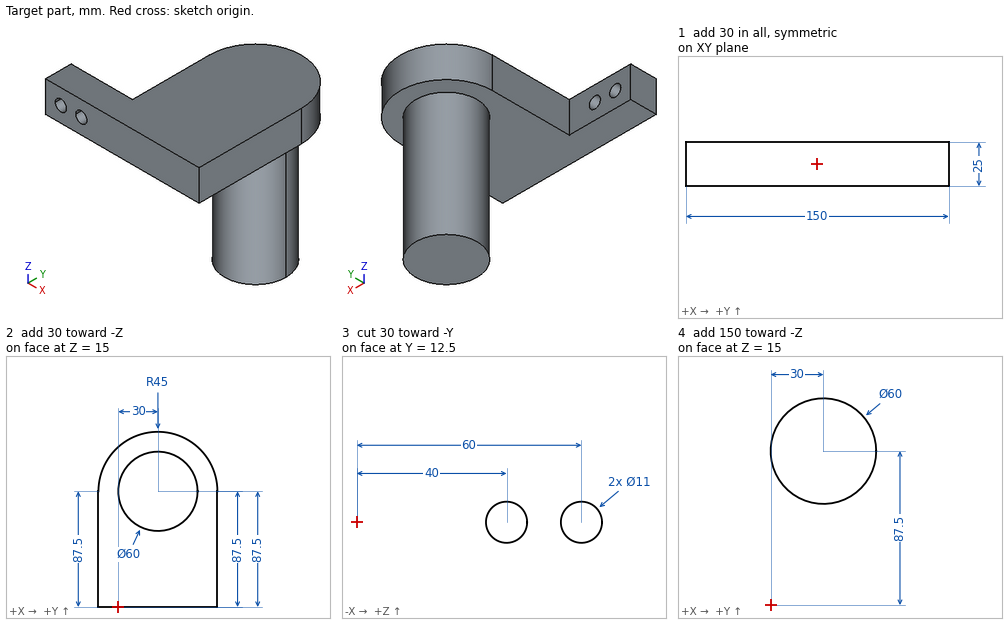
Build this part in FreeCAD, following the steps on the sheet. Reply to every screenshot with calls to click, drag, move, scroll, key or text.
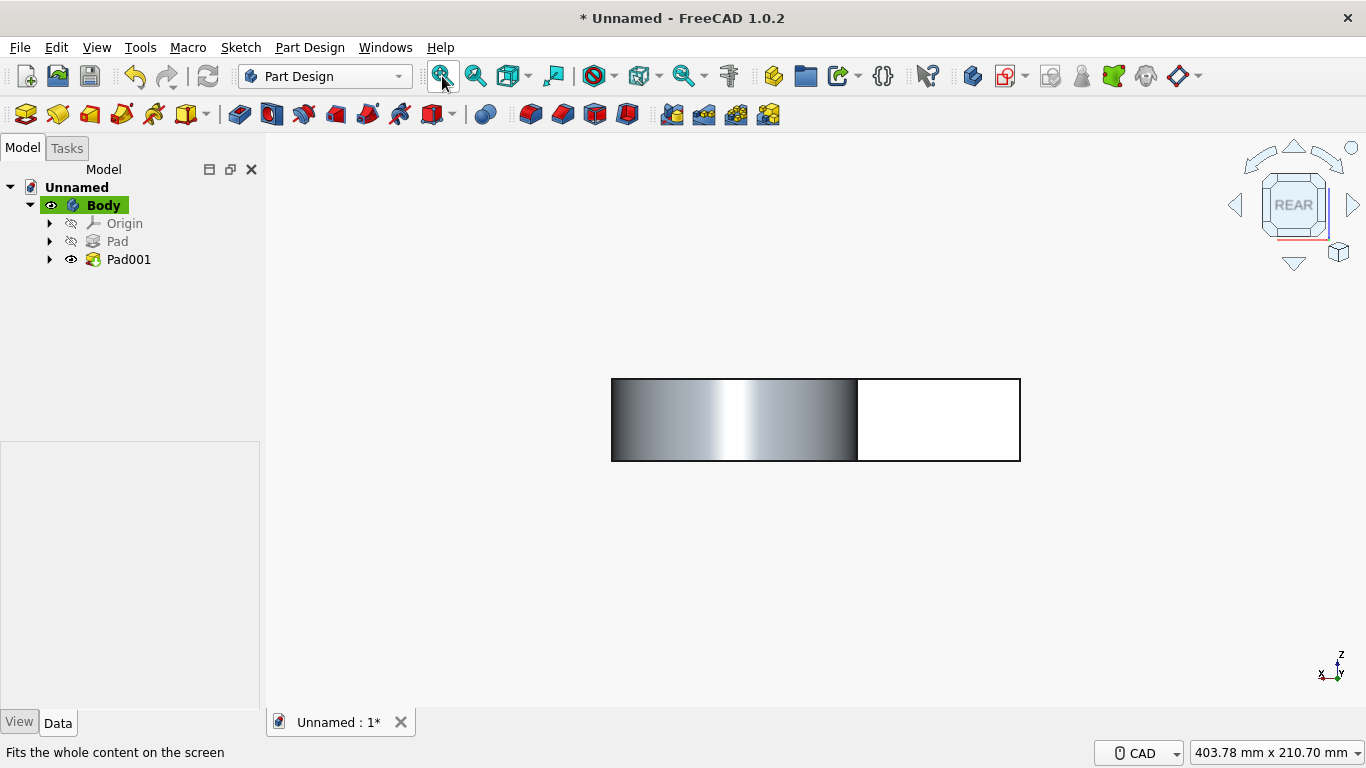
click(915, 419)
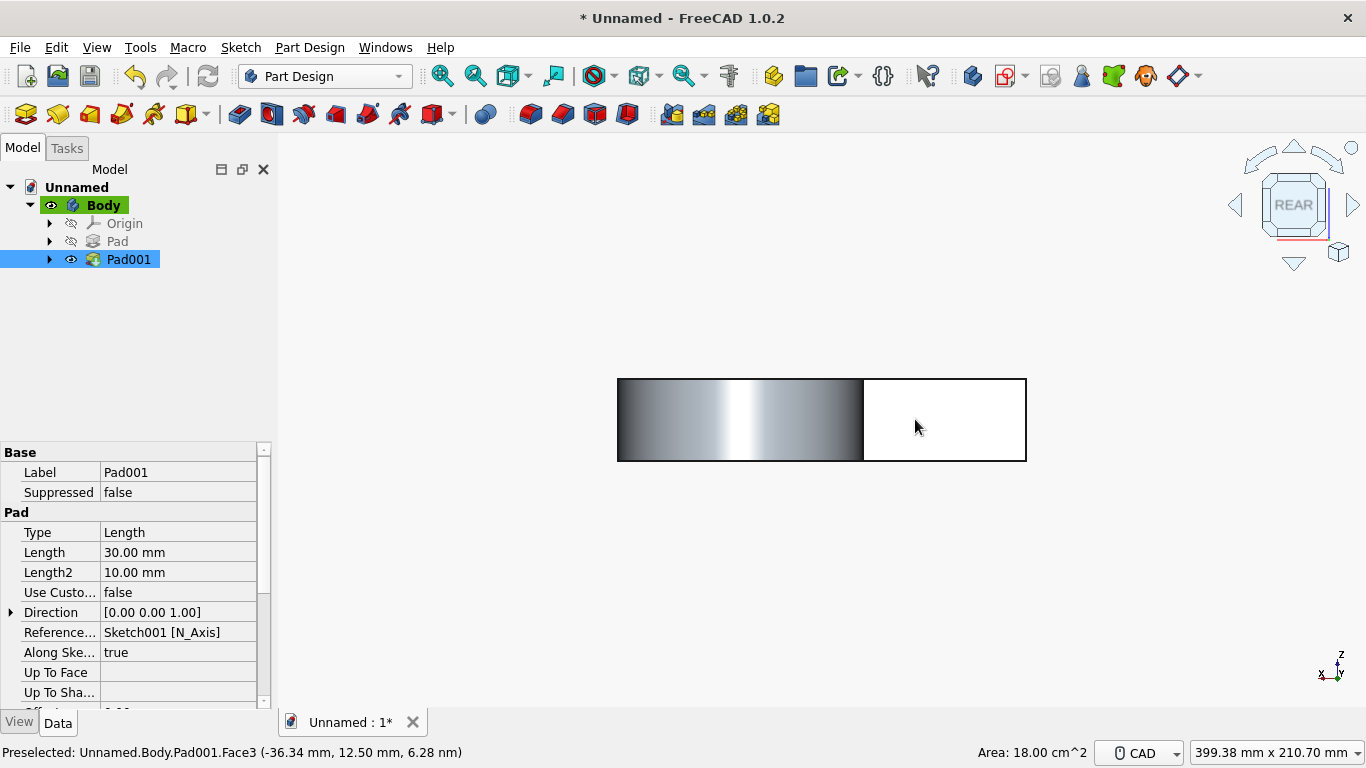
click(1006, 76)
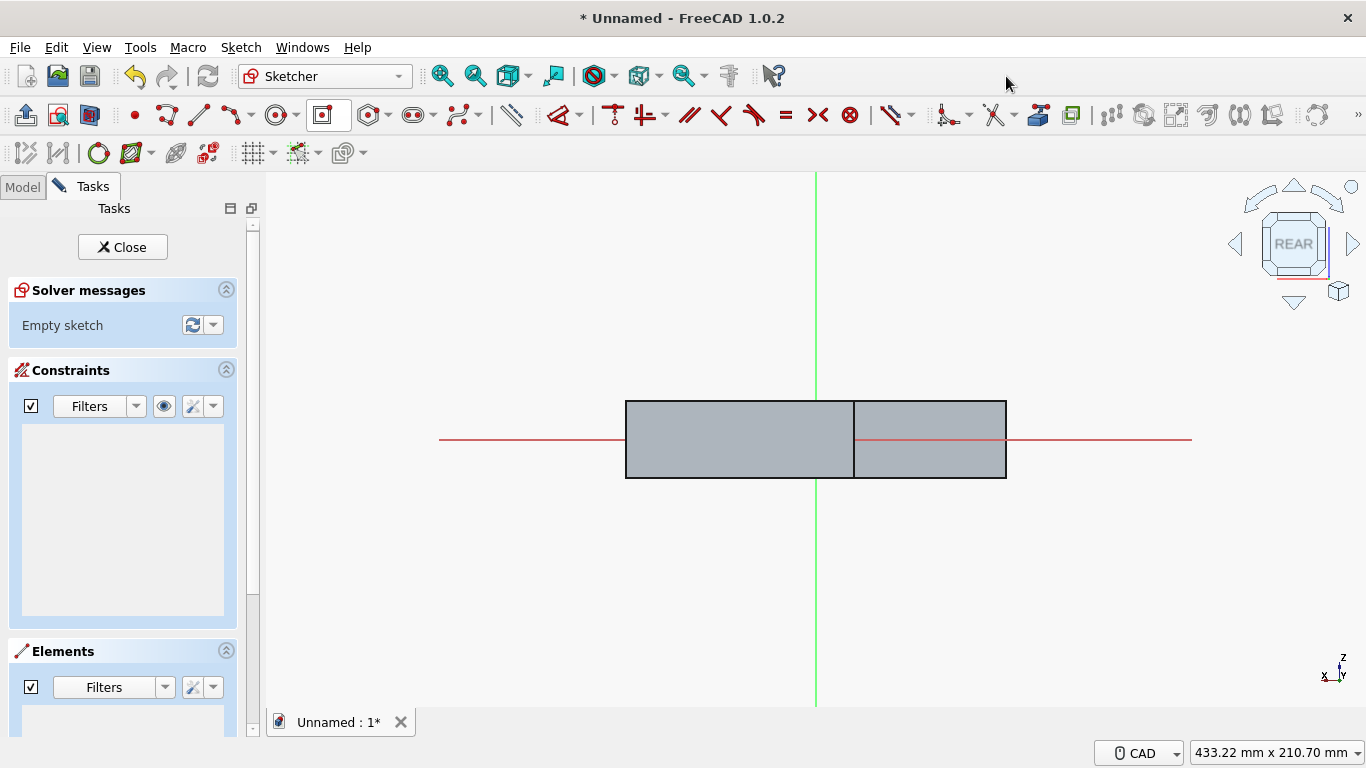
scroll(949, 440, up, 7)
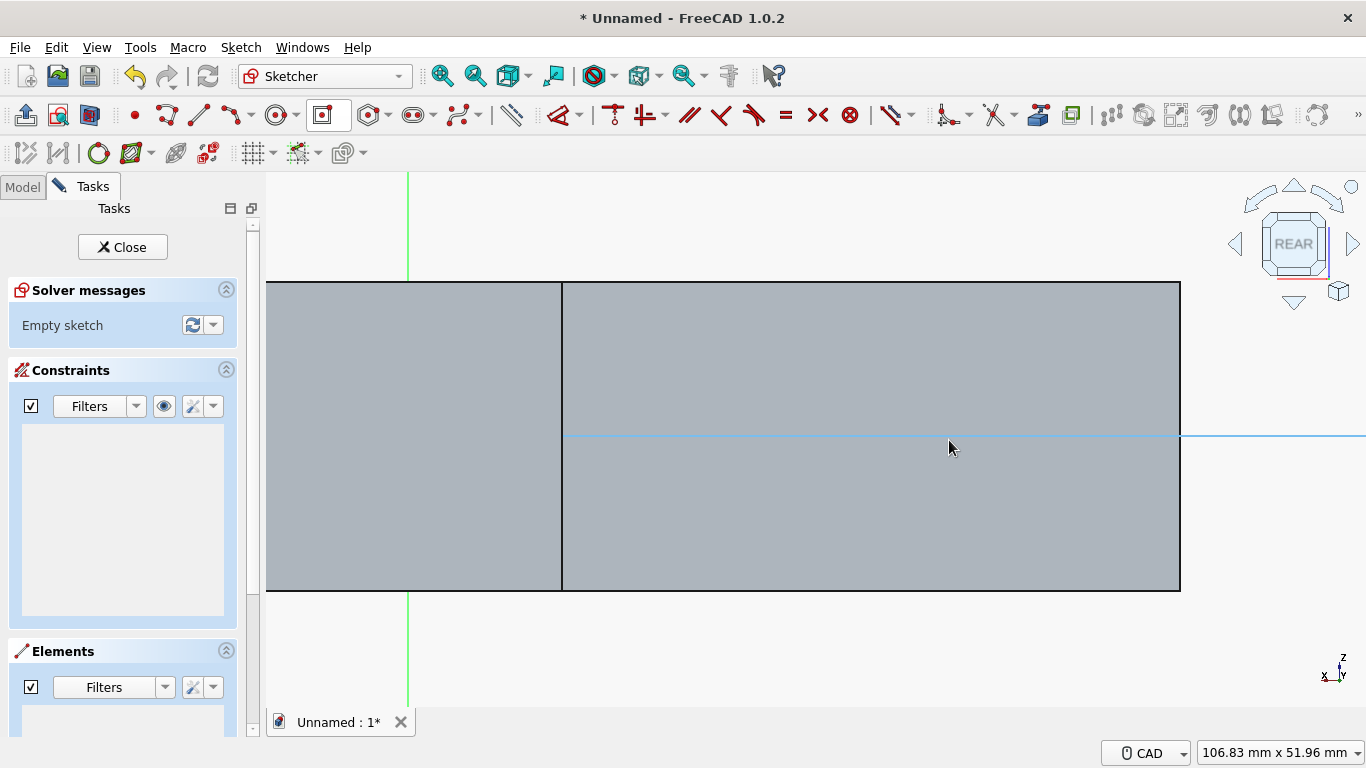
key(g)
key(c)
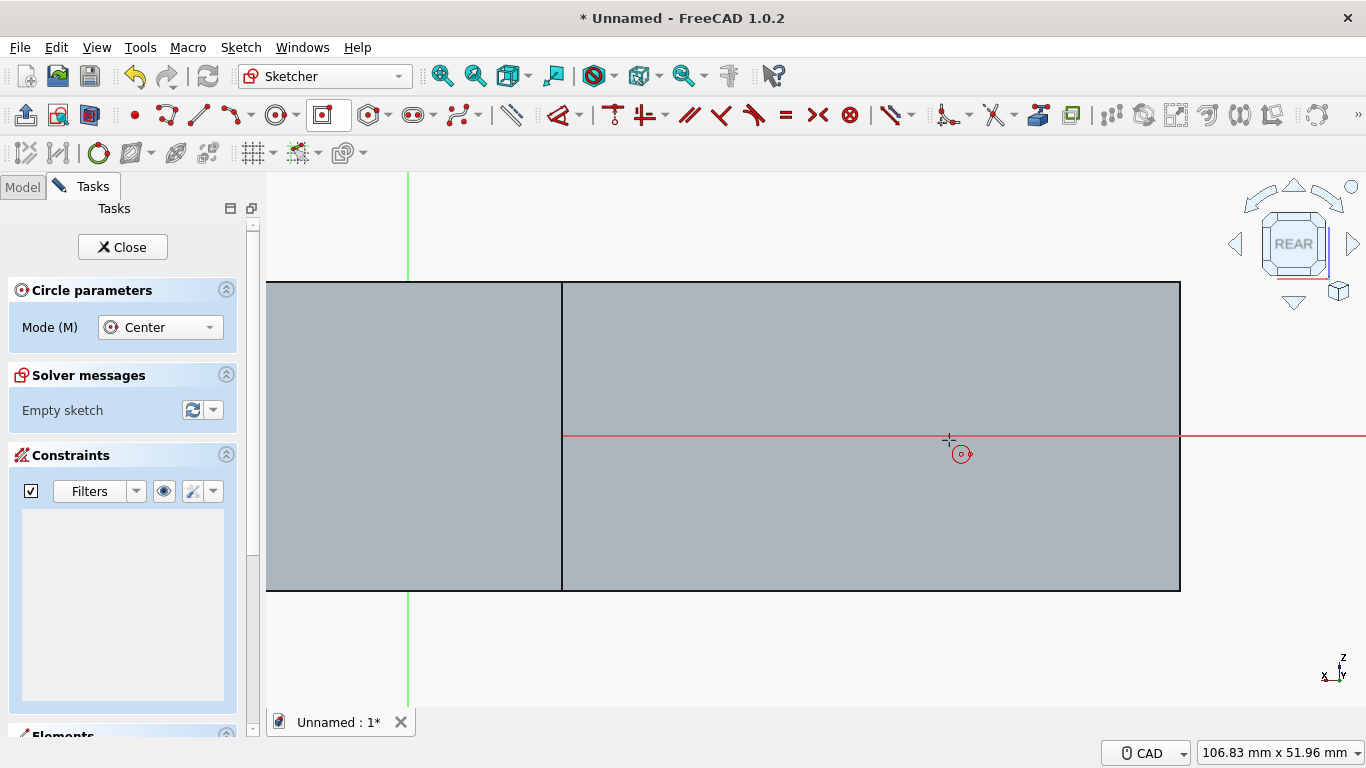
click(1026, 436)
click(1066, 396)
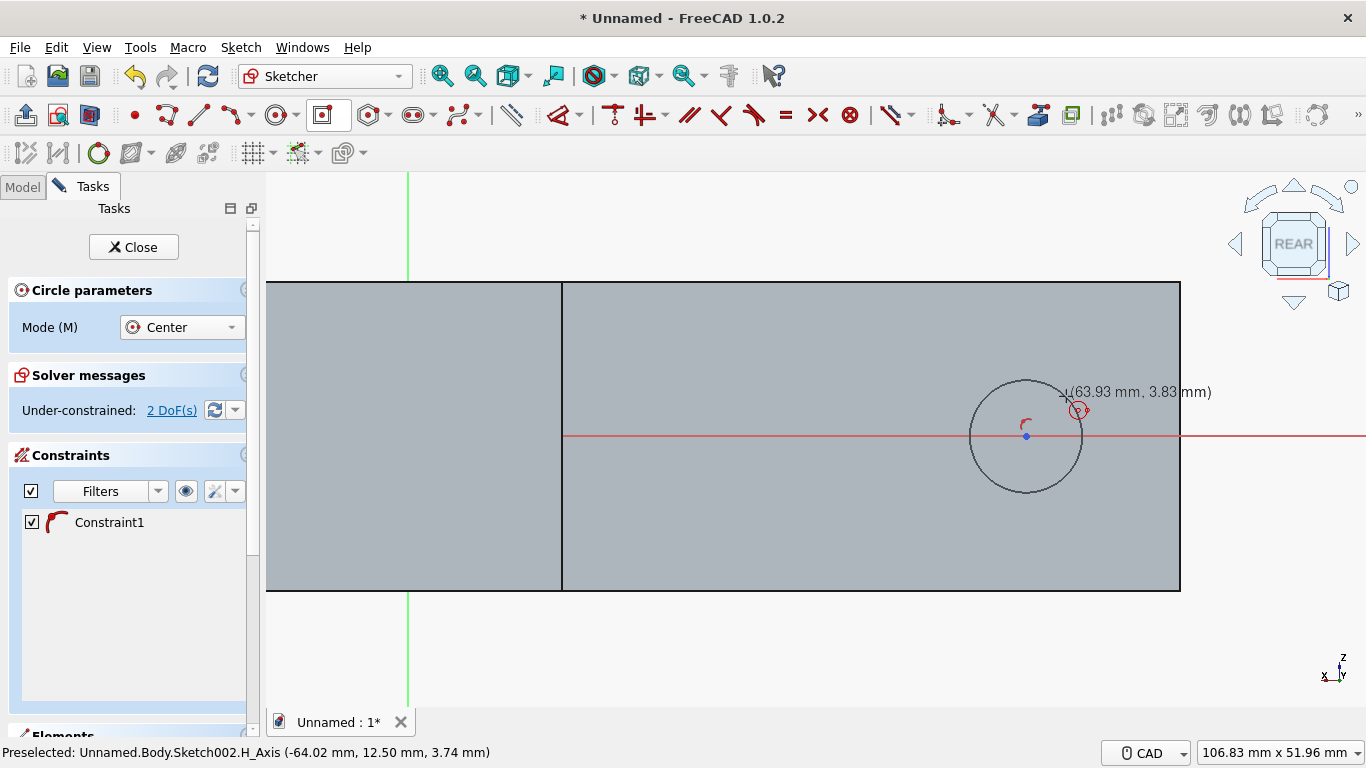
click(820, 436)
click(860, 396)
key(Escape)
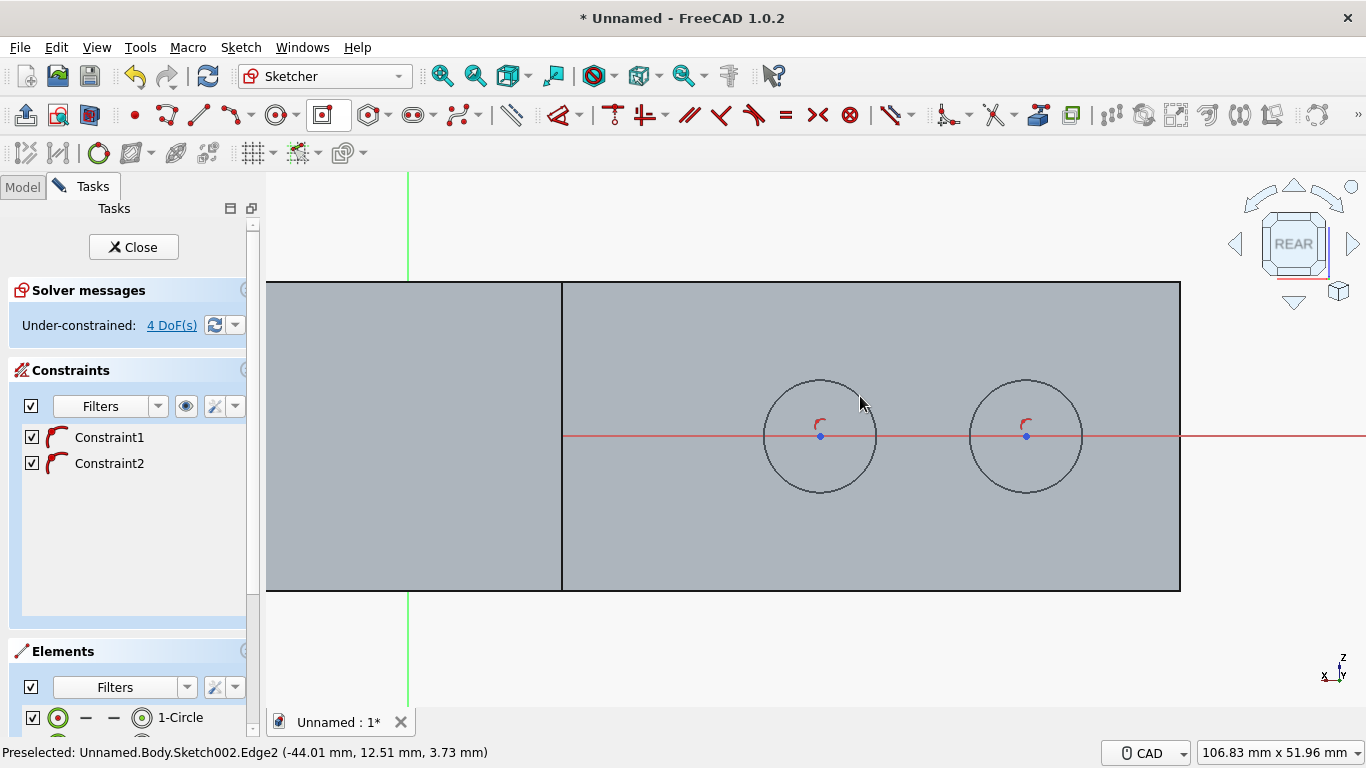
click(1066, 397)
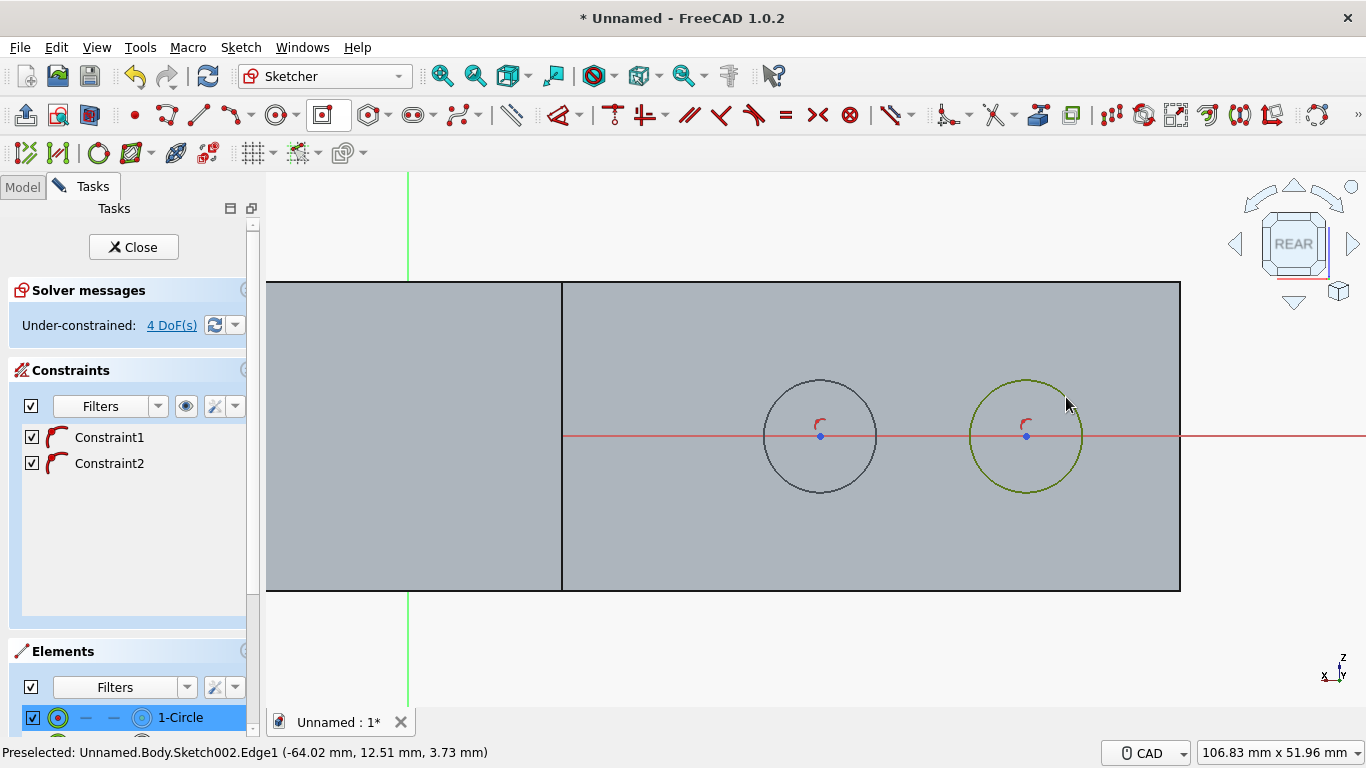
click(860, 397)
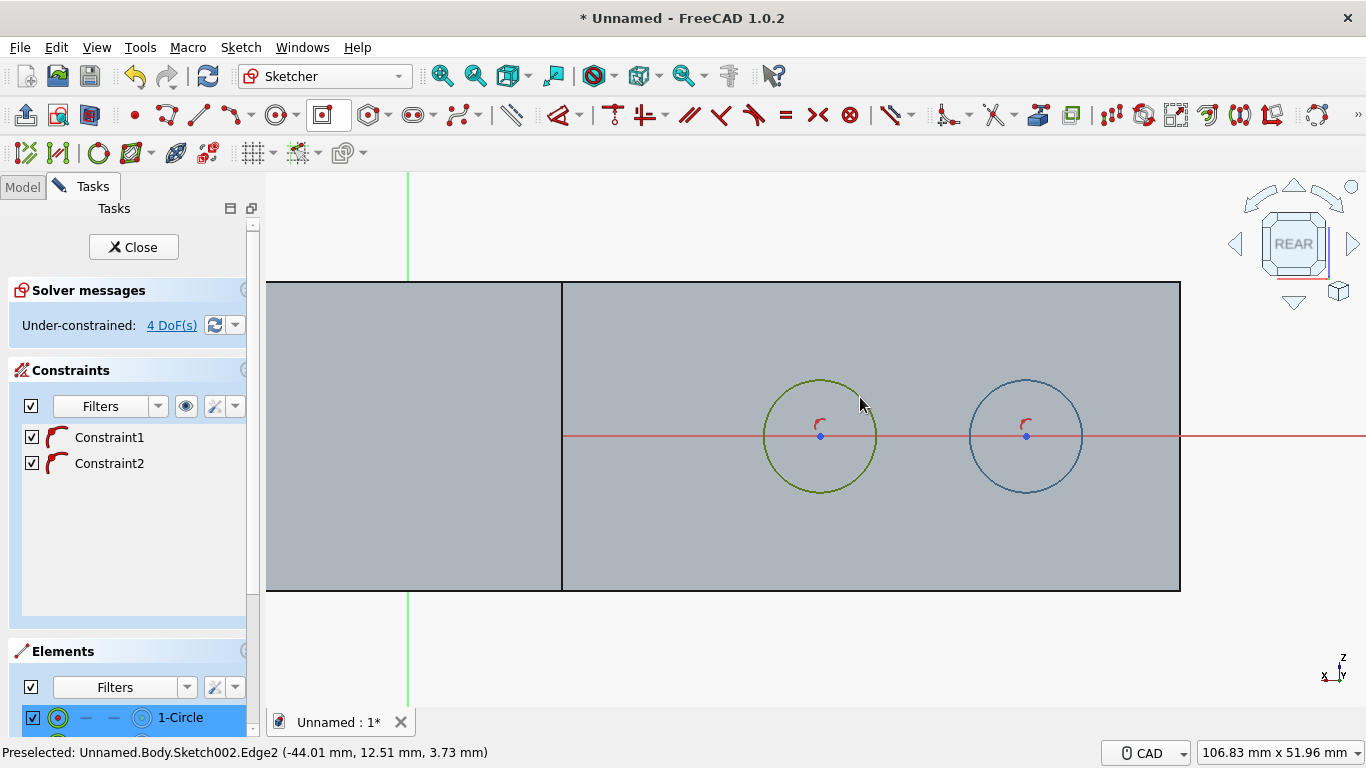
click(786, 116)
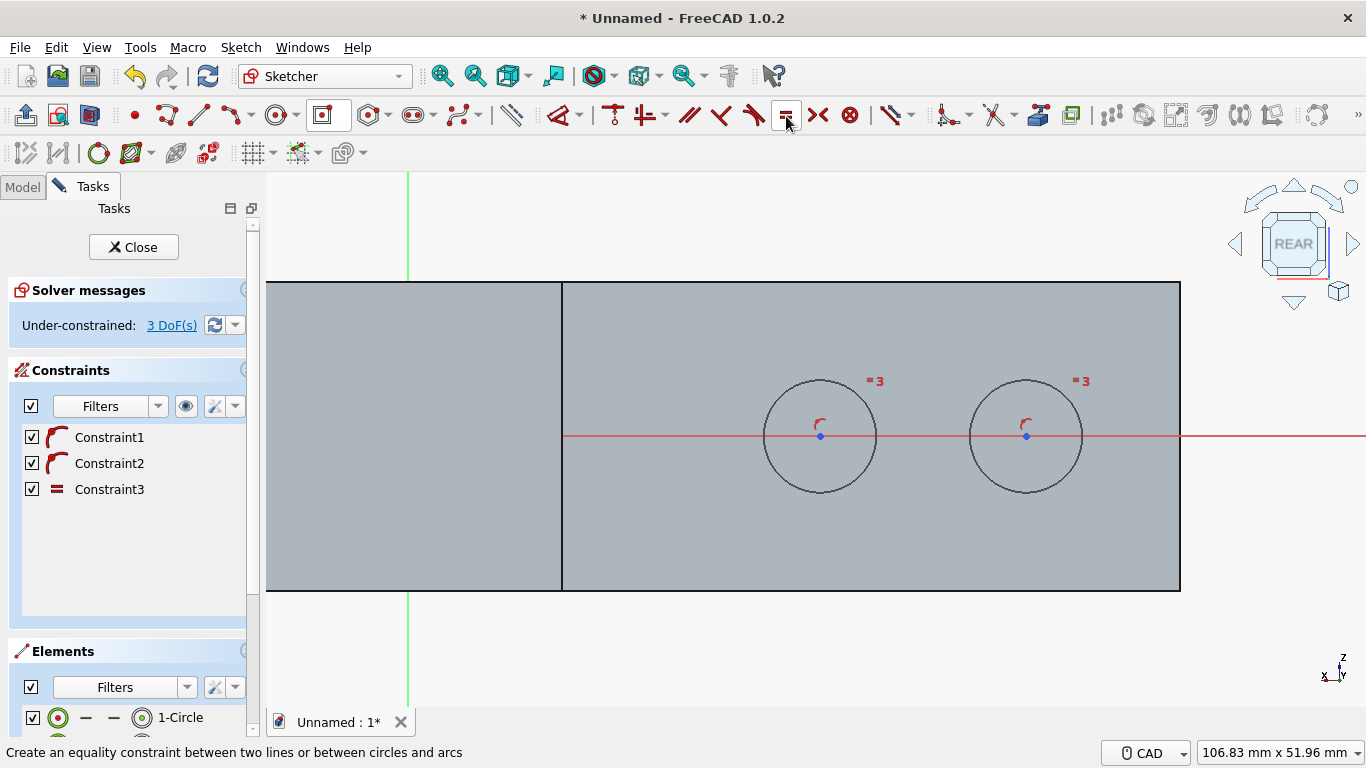
click(558, 116)